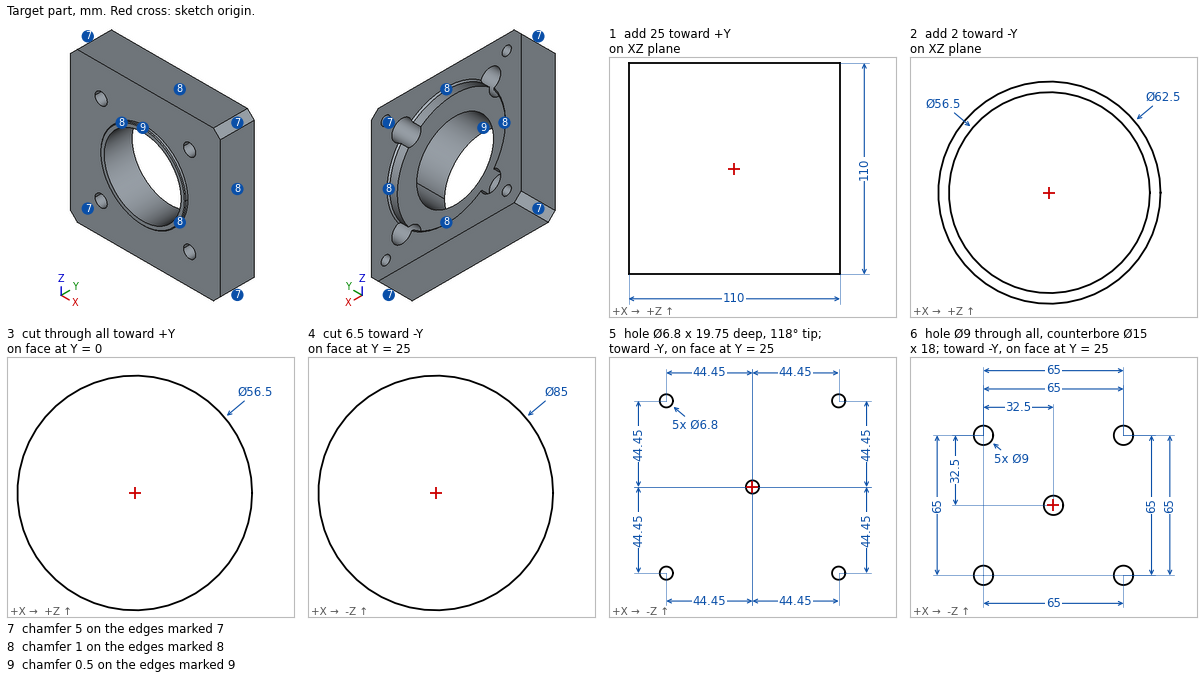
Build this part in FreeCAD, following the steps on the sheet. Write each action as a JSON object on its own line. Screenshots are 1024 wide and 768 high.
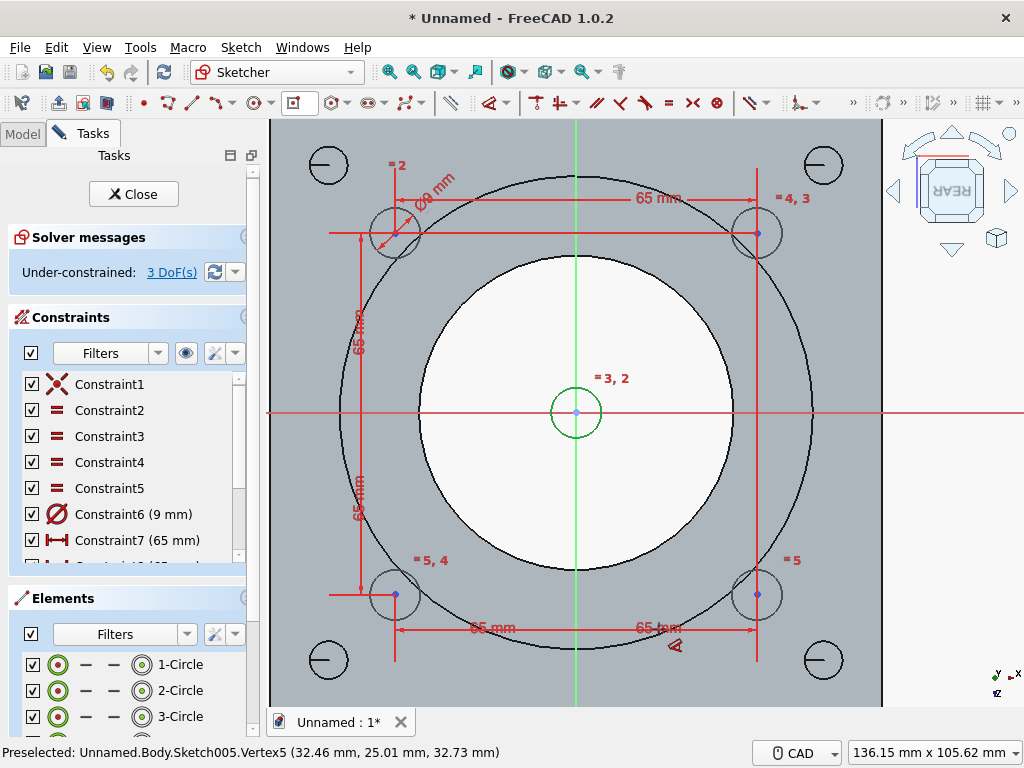
{"action": "left_click", "coordinate": [757, 233]}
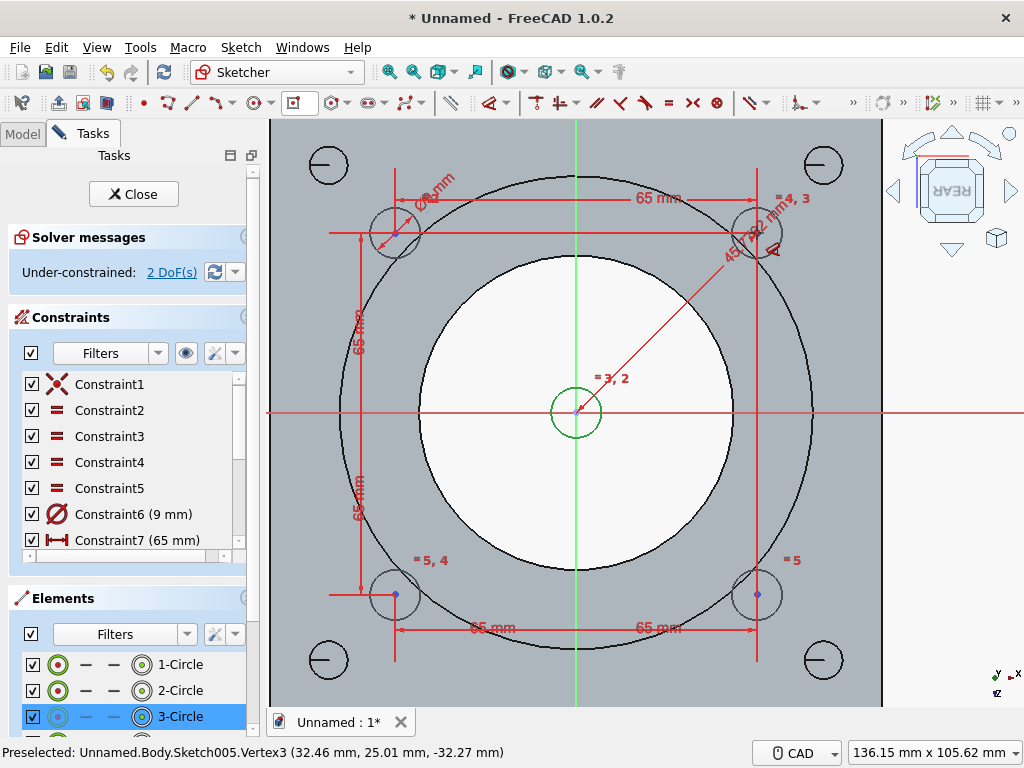
{"action": "left_click", "coordinate": [757, 595]}
{"action": "left_click", "coordinate": [791, 331]}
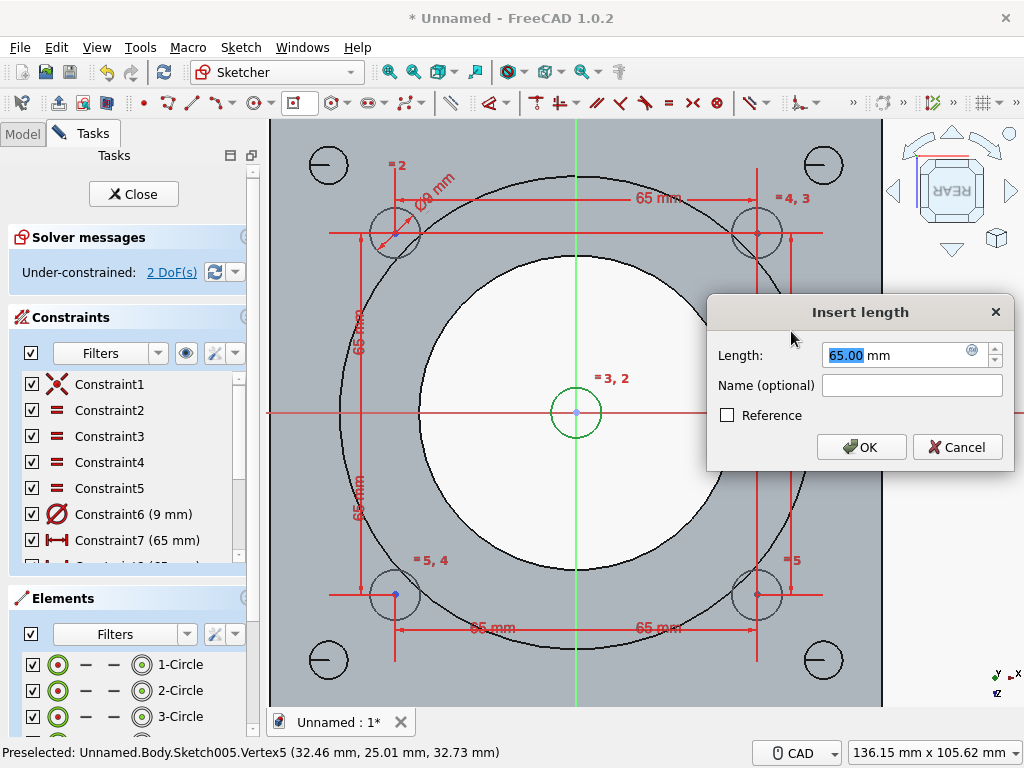
{"action": "type", "text": "65"}
{"action": "key", "text": "Return"}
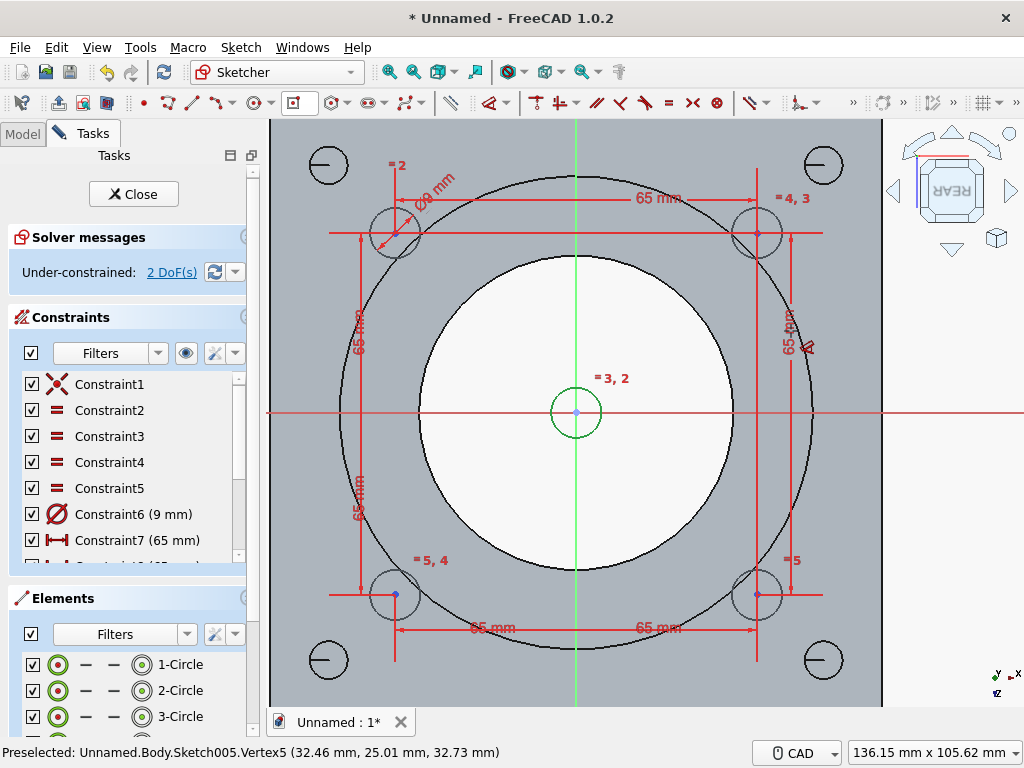
{"action": "left_click", "coordinate": [395, 233]}
{"action": "left_click", "coordinate": [527, 199]}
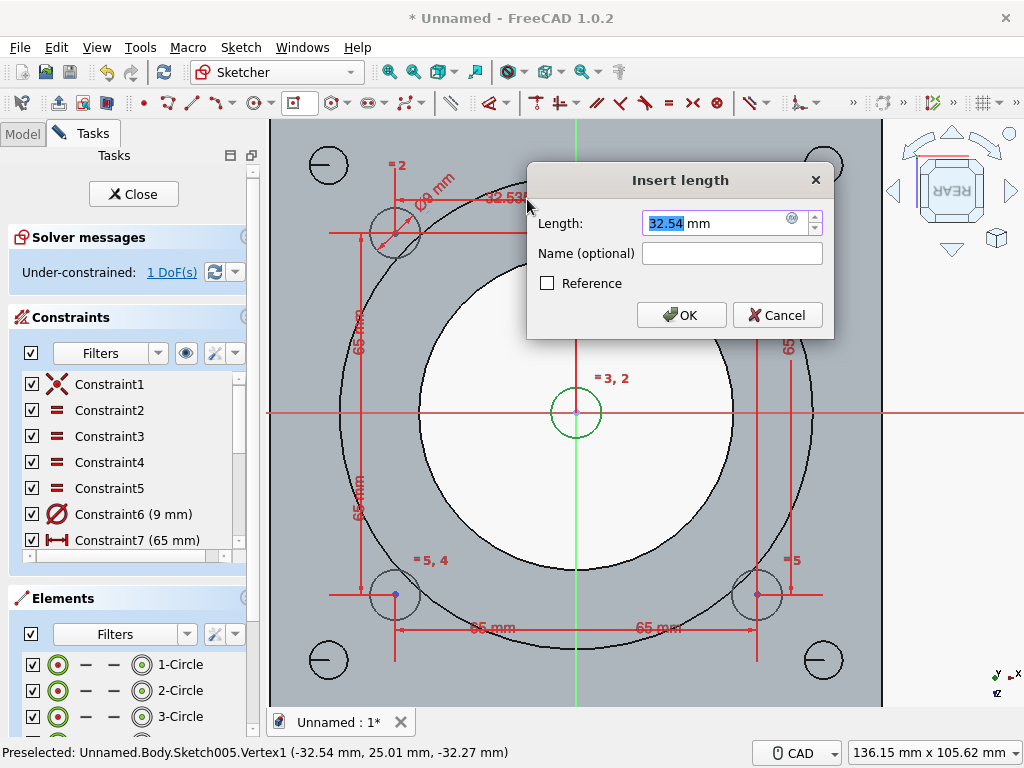
{"action": "type", "text": "32.5"}
{"action": "key", "text": "Return"}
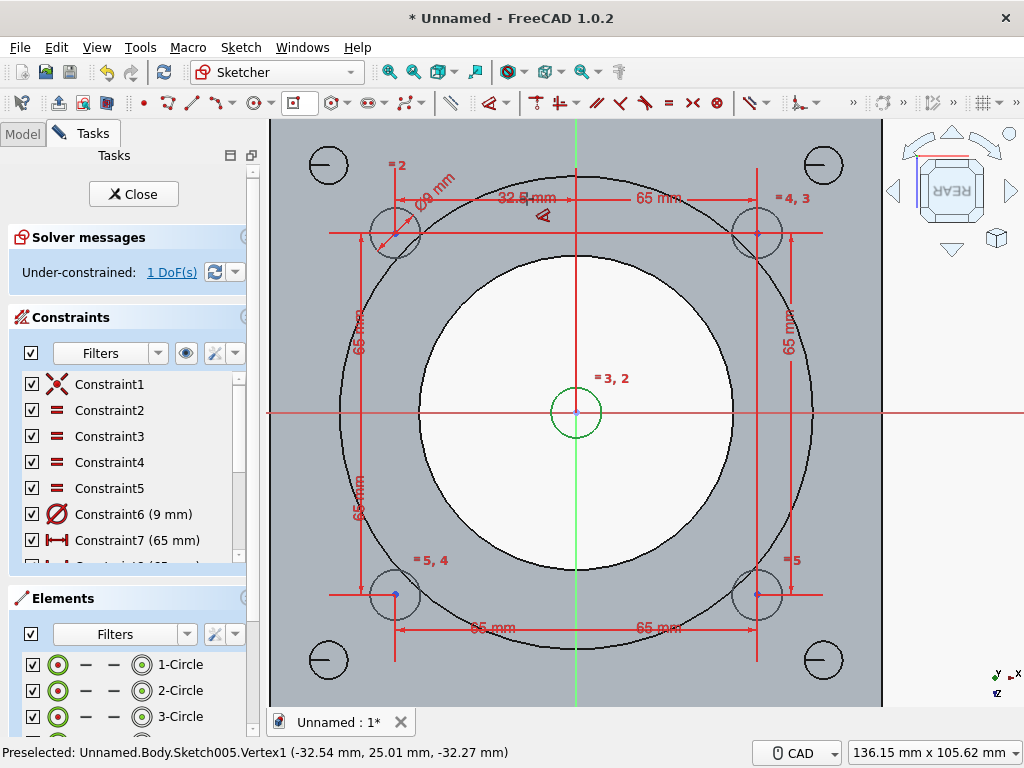
{"action": "left_click", "coordinate": [395, 233]}
{"action": "left_click", "coordinate": [361, 282]}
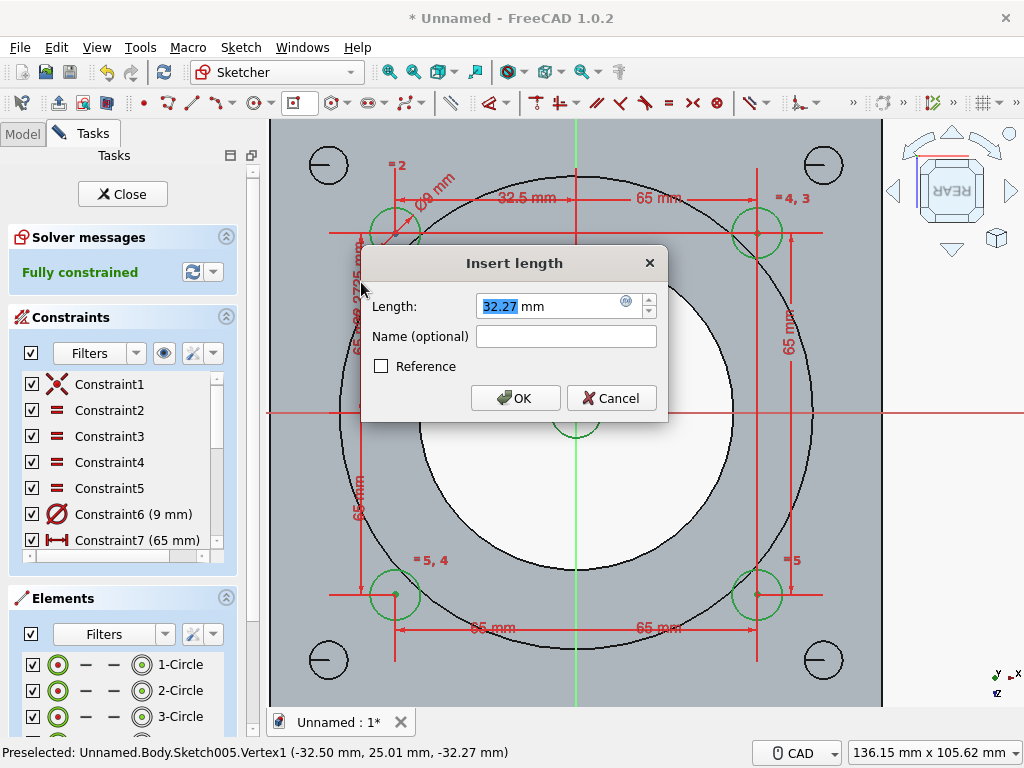
{"action": "type", "text": "32.5"}
{"action": "key", "text": "Return"}
{"action": "key", "text": "Escape"}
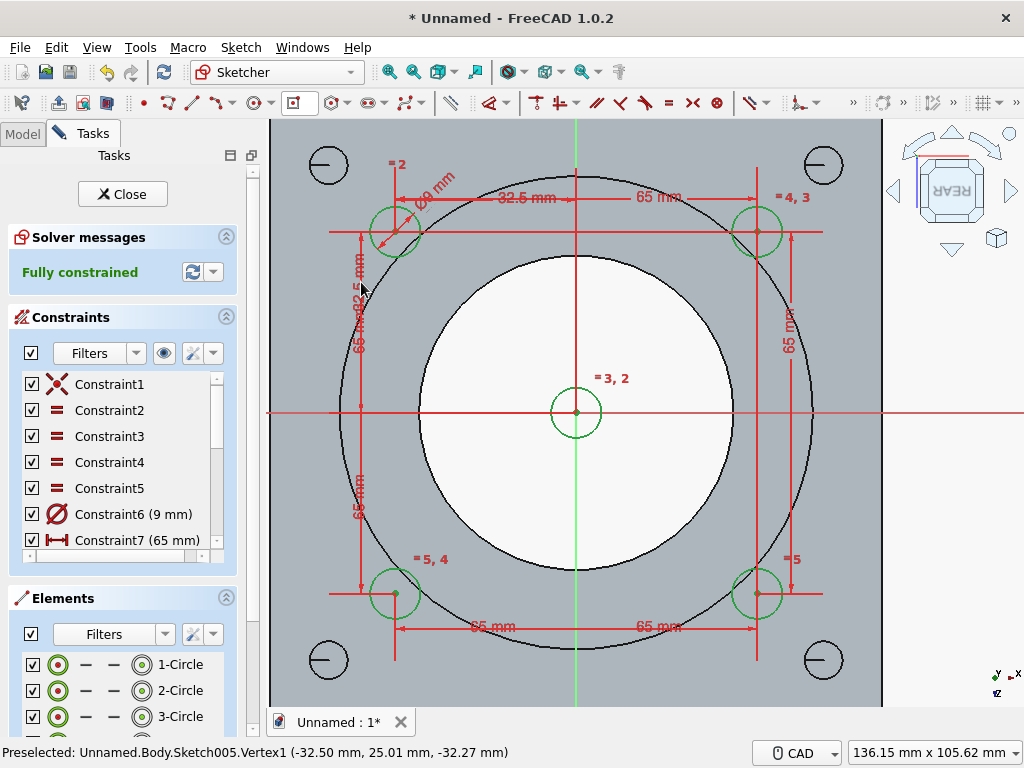
{"action": "left_click", "coordinate": [123, 194]}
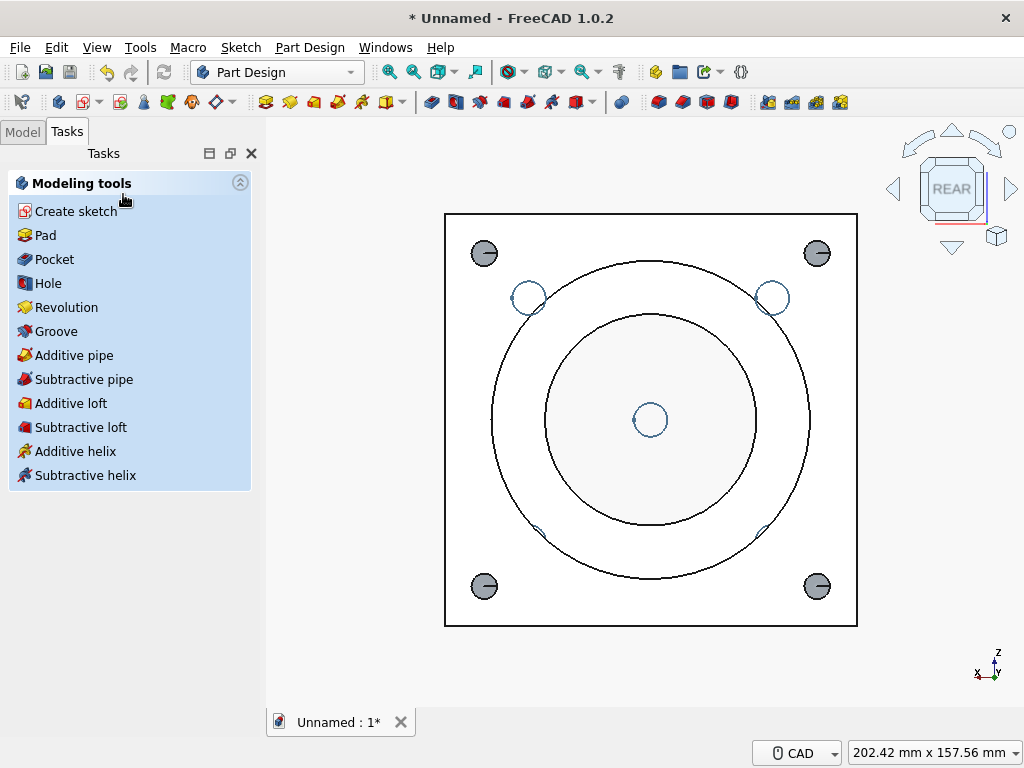
{"action": "left_click", "coordinate": [456, 102]}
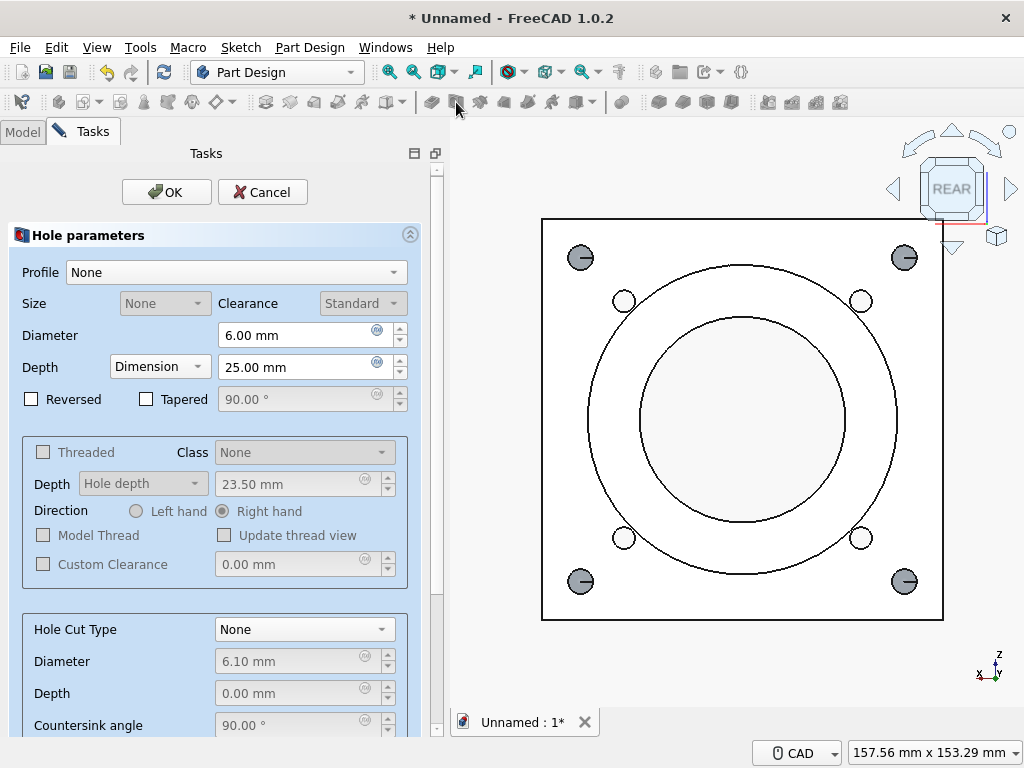
{"action": "triple_click", "coordinate": [305, 335]}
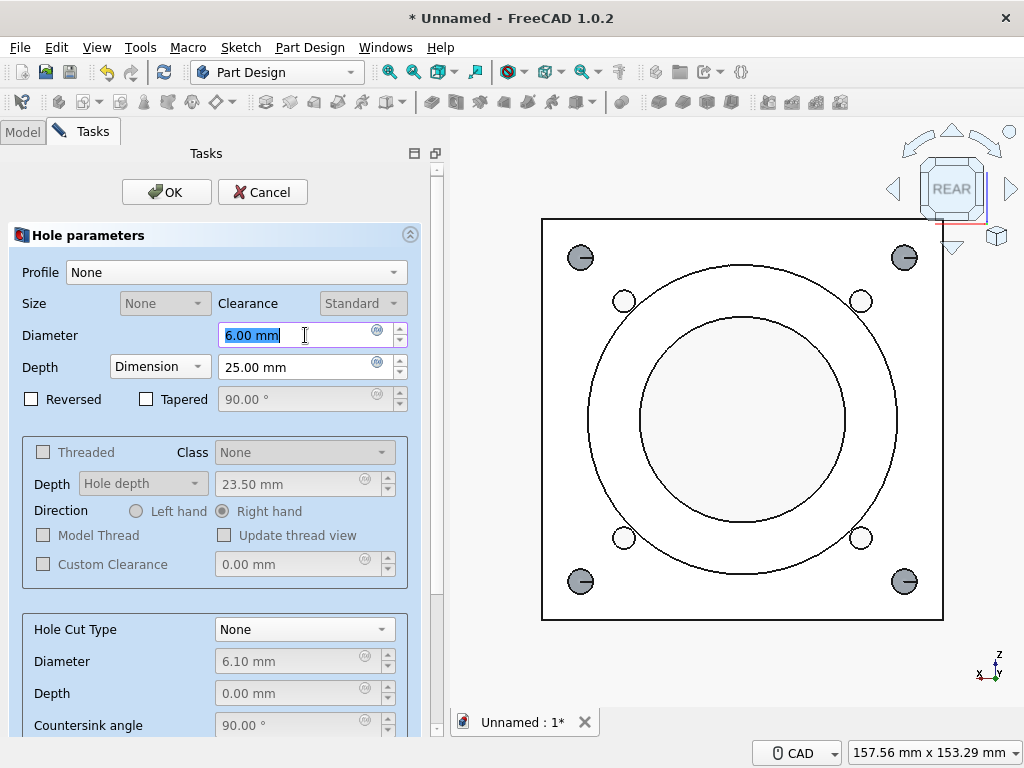
{"action": "type", "text": "9"}
{"action": "key", "text": "Tab"}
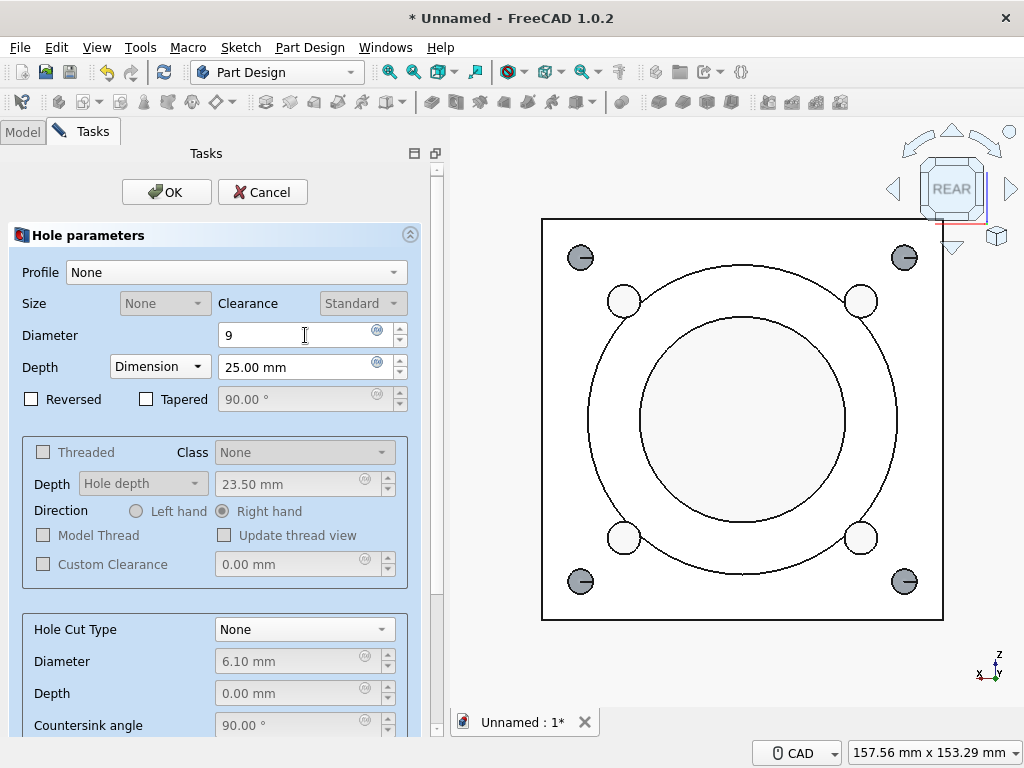
{"action": "left_click", "coordinate": [161, 366]}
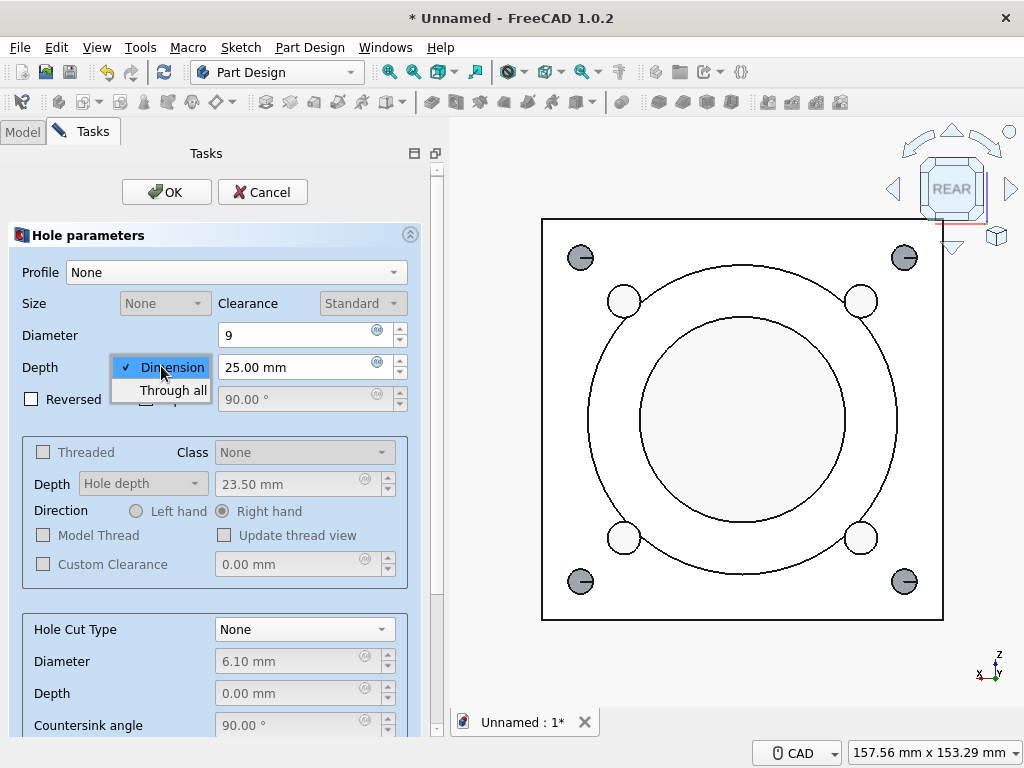
{"action": "left_click", "coordinate": [160, 390]}